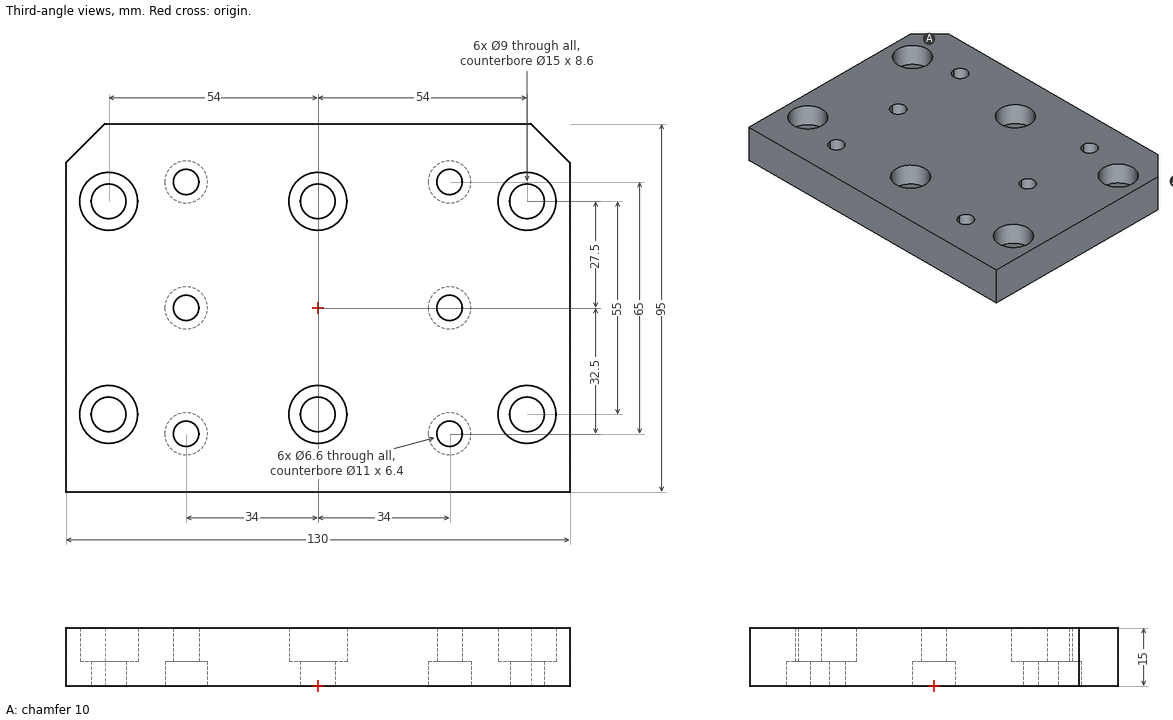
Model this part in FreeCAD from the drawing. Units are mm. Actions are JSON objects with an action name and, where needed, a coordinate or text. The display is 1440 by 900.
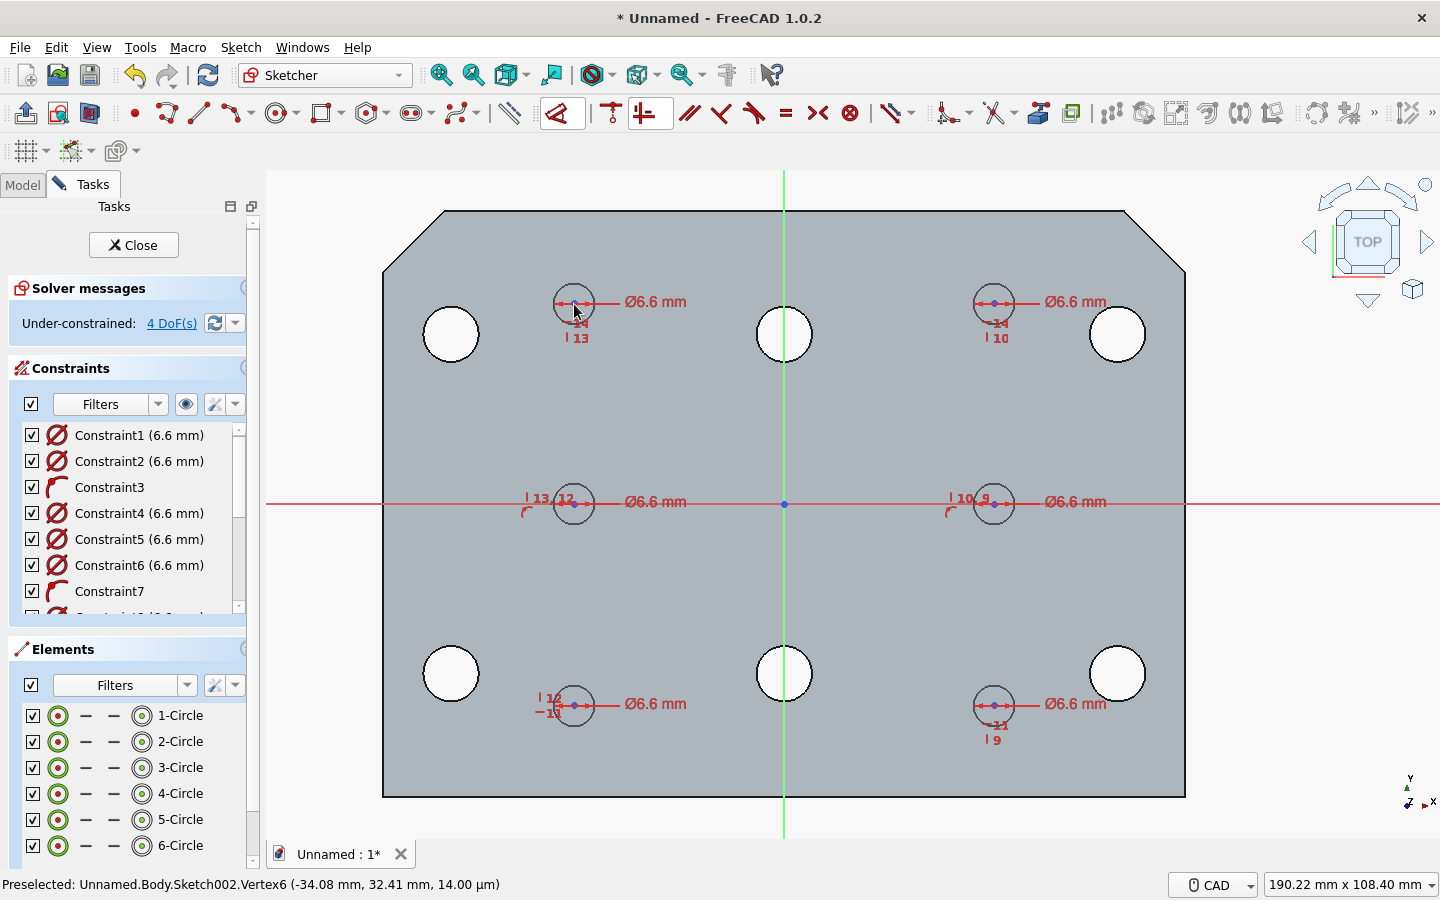
{"action": "key", "text": "d"}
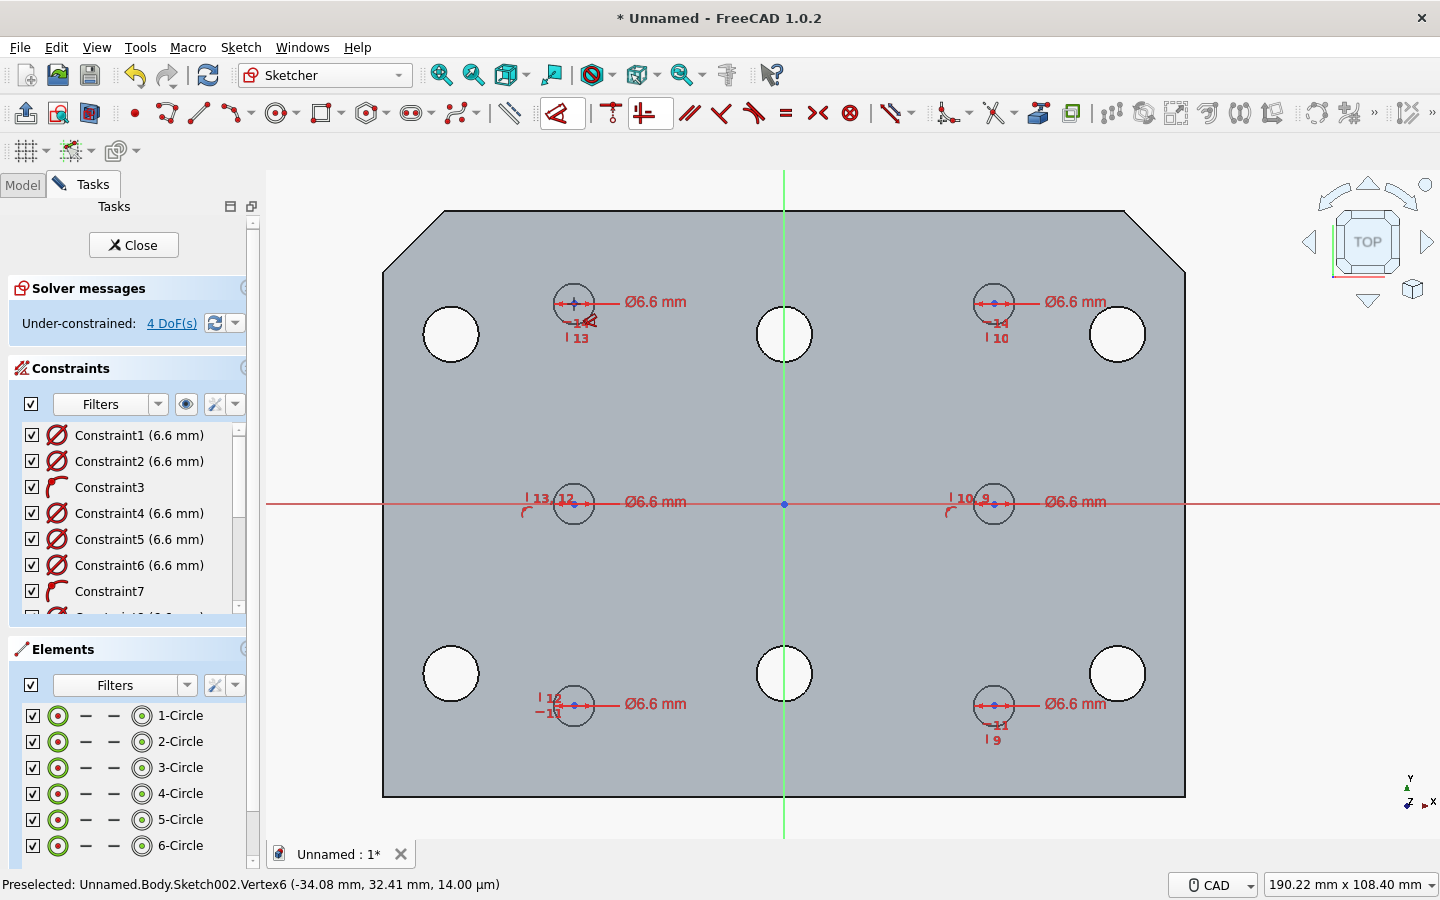
{"action": "left_click", "coordinate": [994, 706]}
{"action": "left_click", "coordinate": [889, 740]}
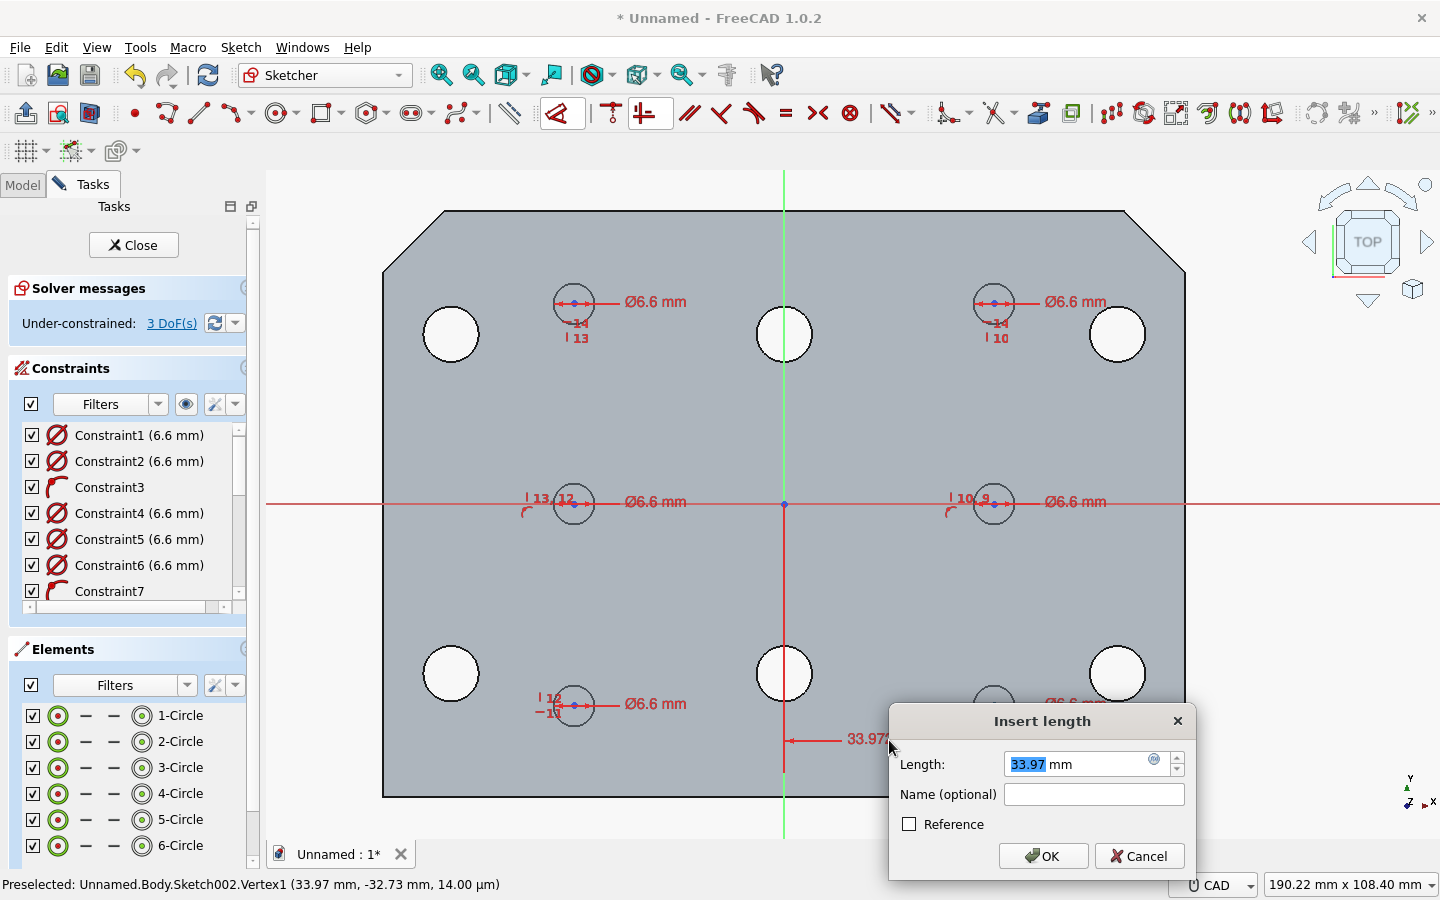
{"action": "type", "text": "34"}
{"action": "key", "text": "Return"}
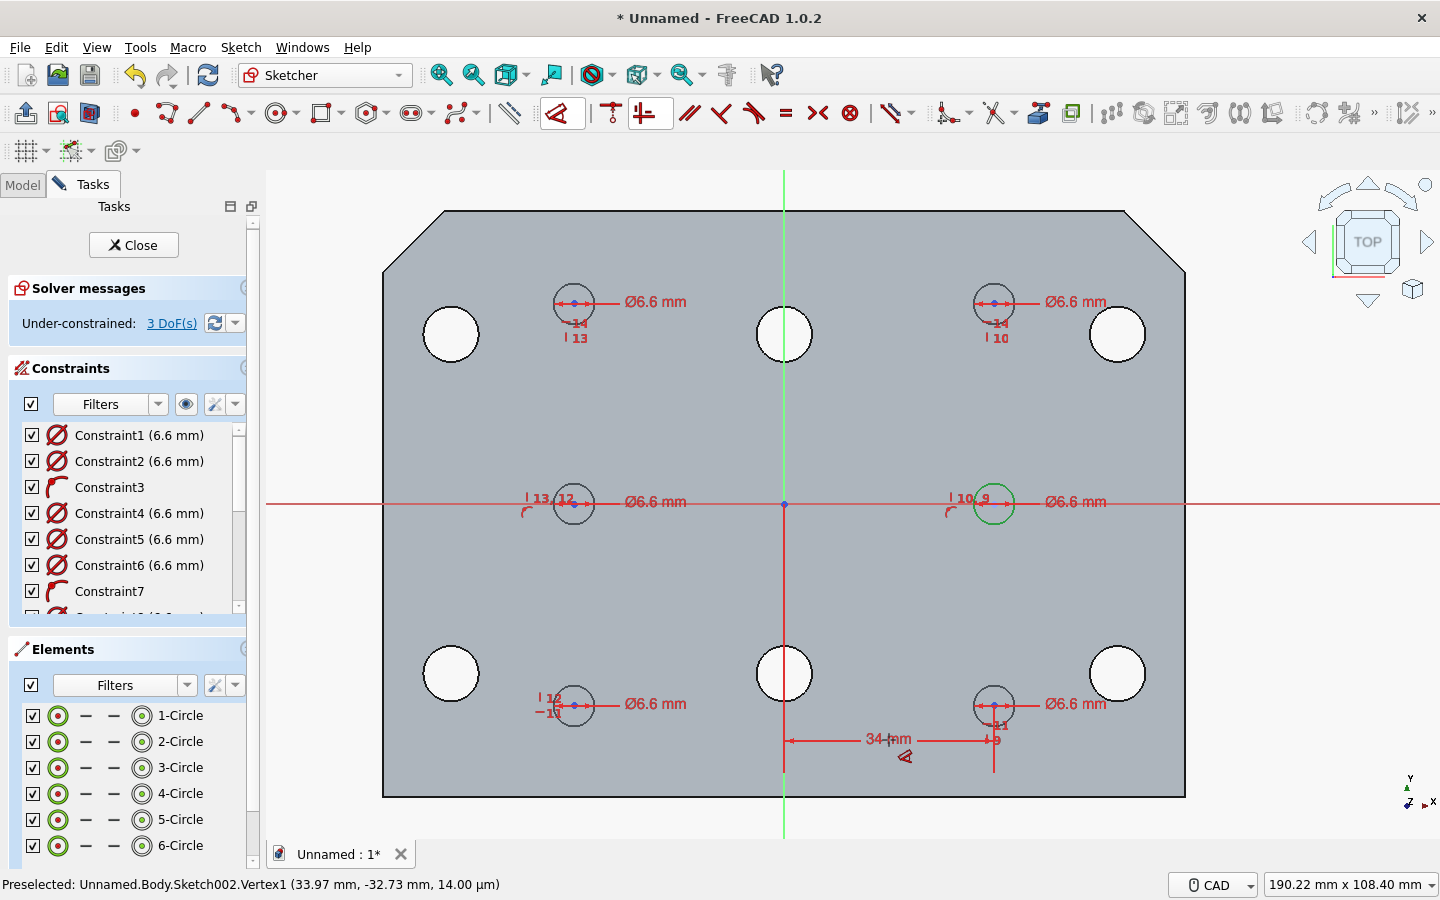
{"action": "left_click", "coordinate": [574, 706]}
{"action": "left_click", "coordinate": [679, 740]}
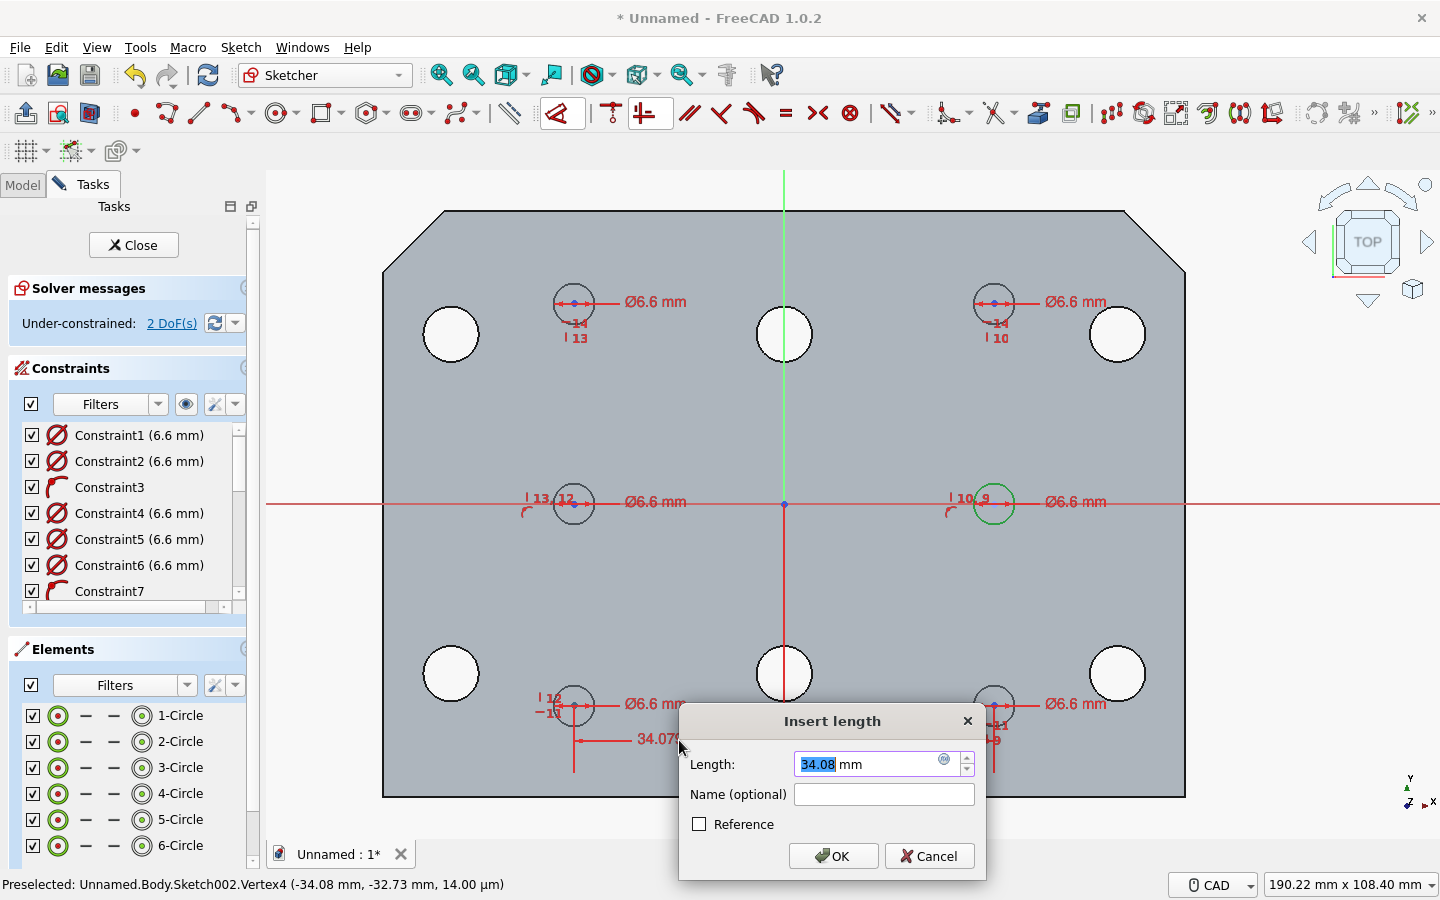
{"action": "type", "text": "34"}
{"action": "key", "text": "Return"}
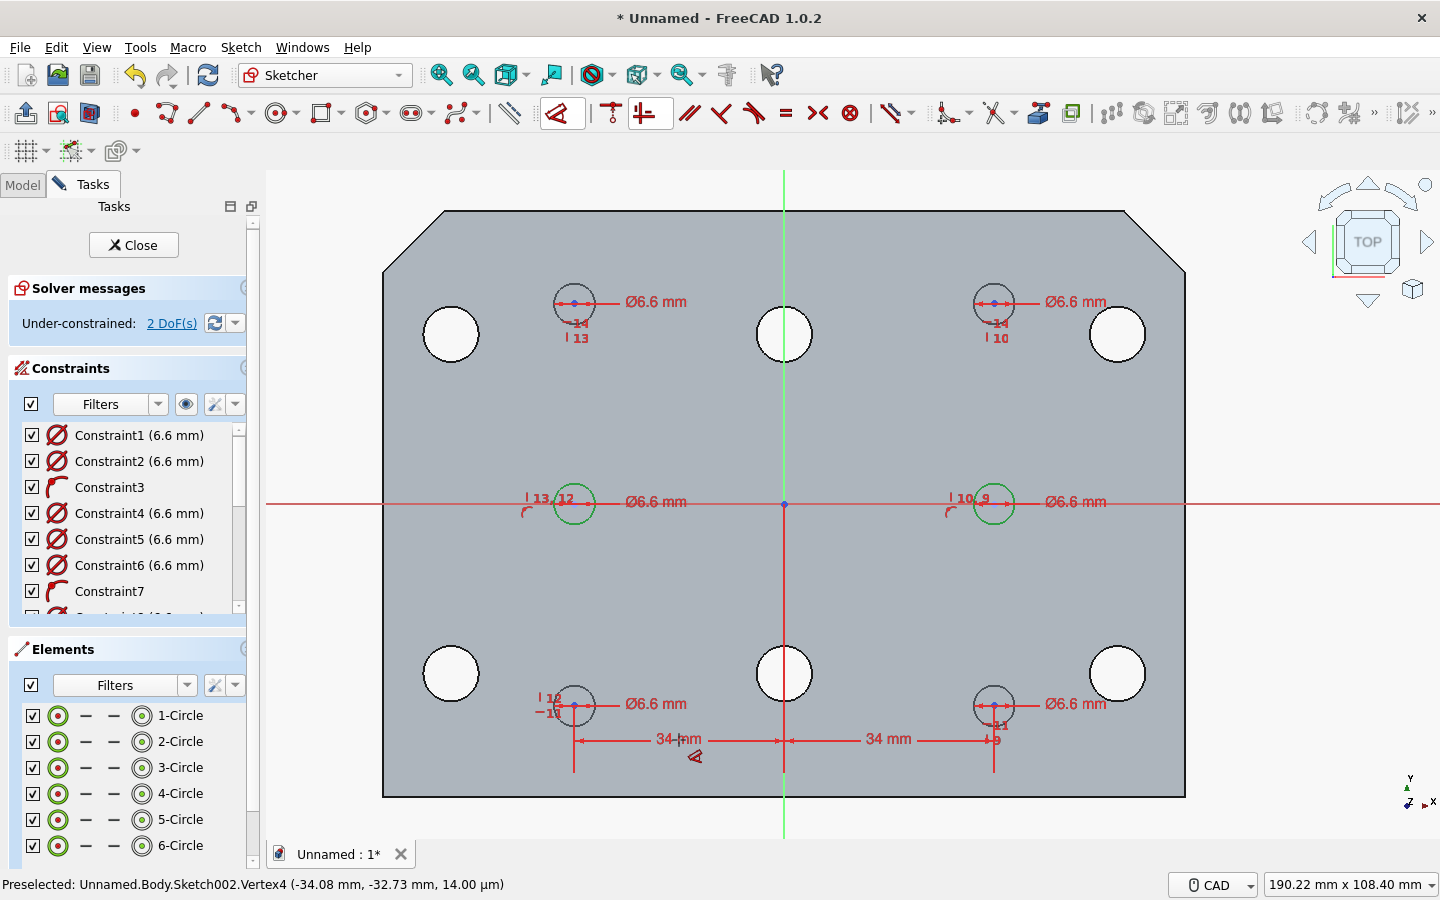
{"action": "left_click", "coordinate": [994, 706]}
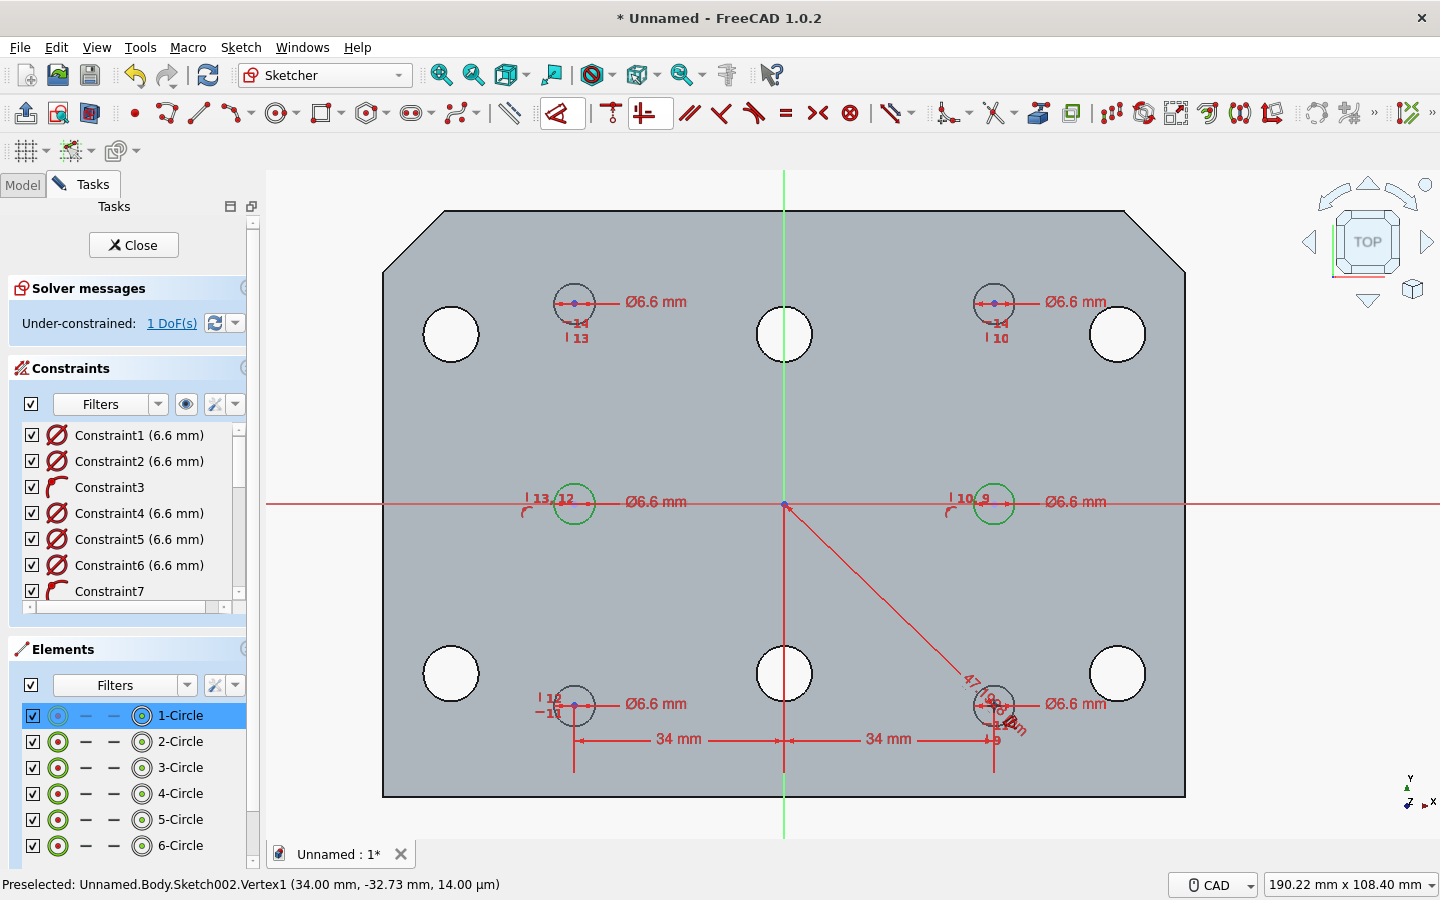
{"action": "left_click", "coordinate": [994, 304]}
{"action": "left_click", "coordinate": [1028, 413]}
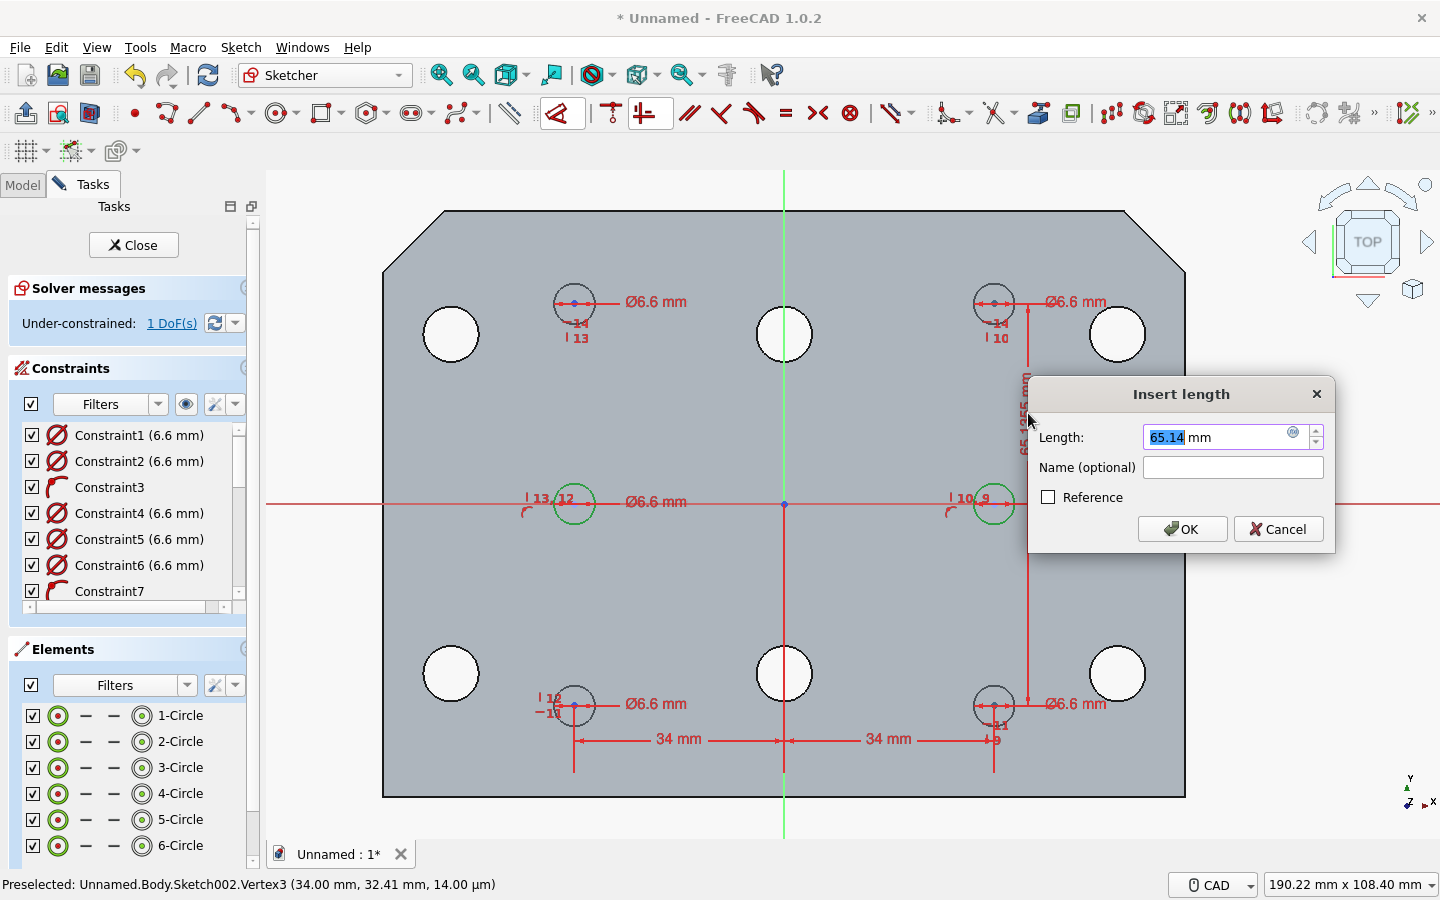
{"action": "type", "text": "65"}
{"action": "key", "text": "Return"}